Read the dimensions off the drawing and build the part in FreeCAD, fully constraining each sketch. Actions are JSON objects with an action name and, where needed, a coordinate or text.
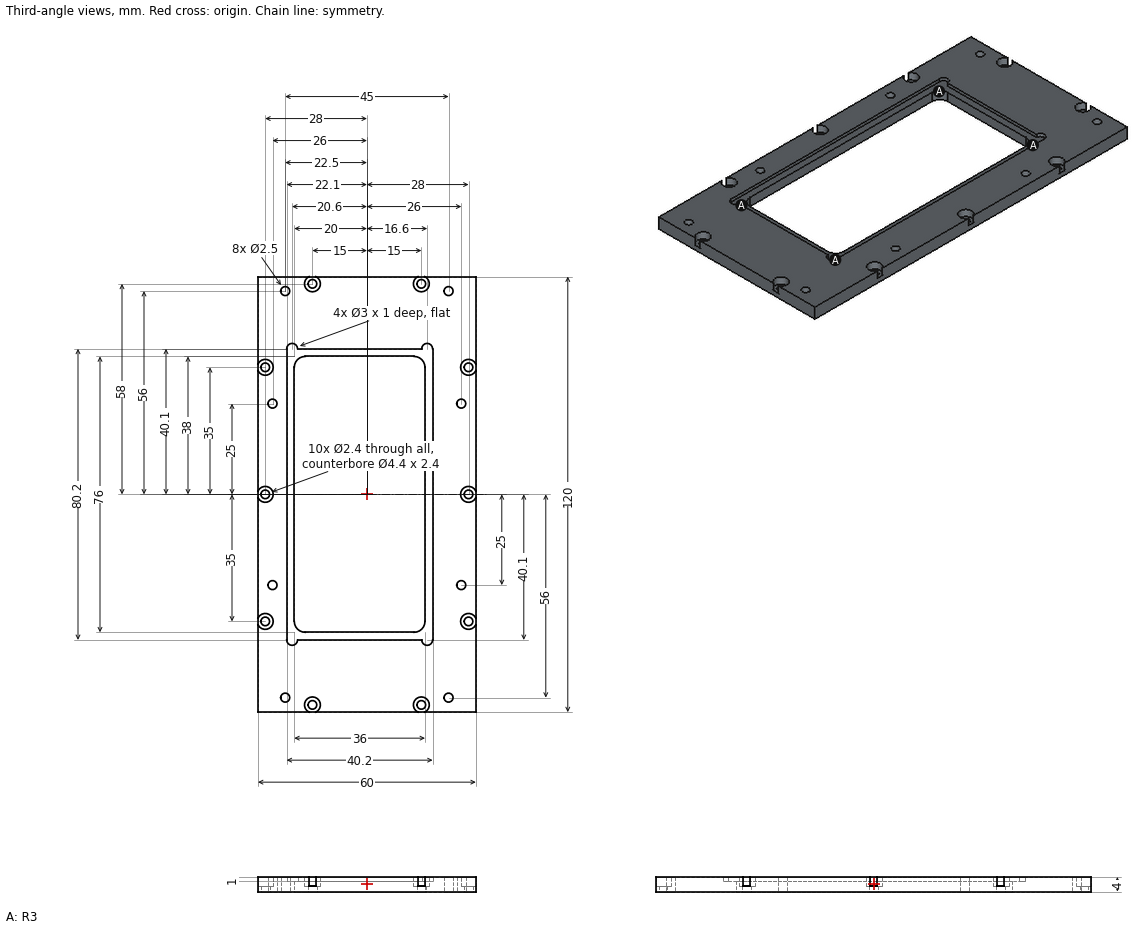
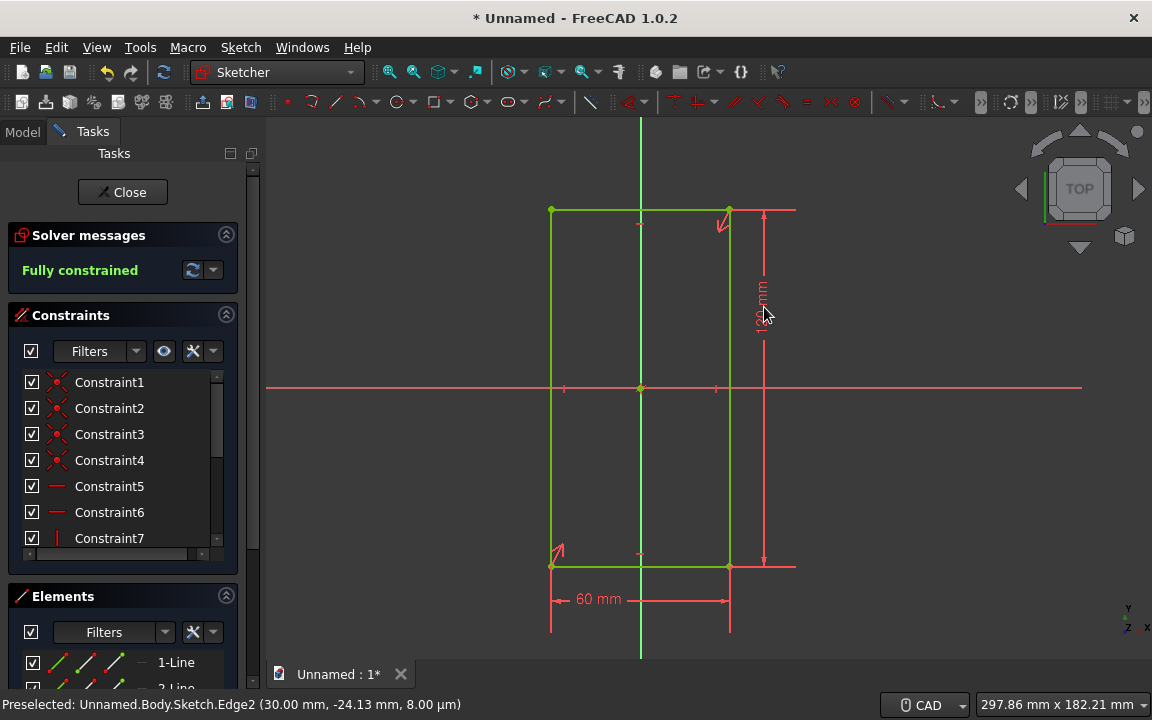
{"action": "left_click", "coordinate": [123, 192]}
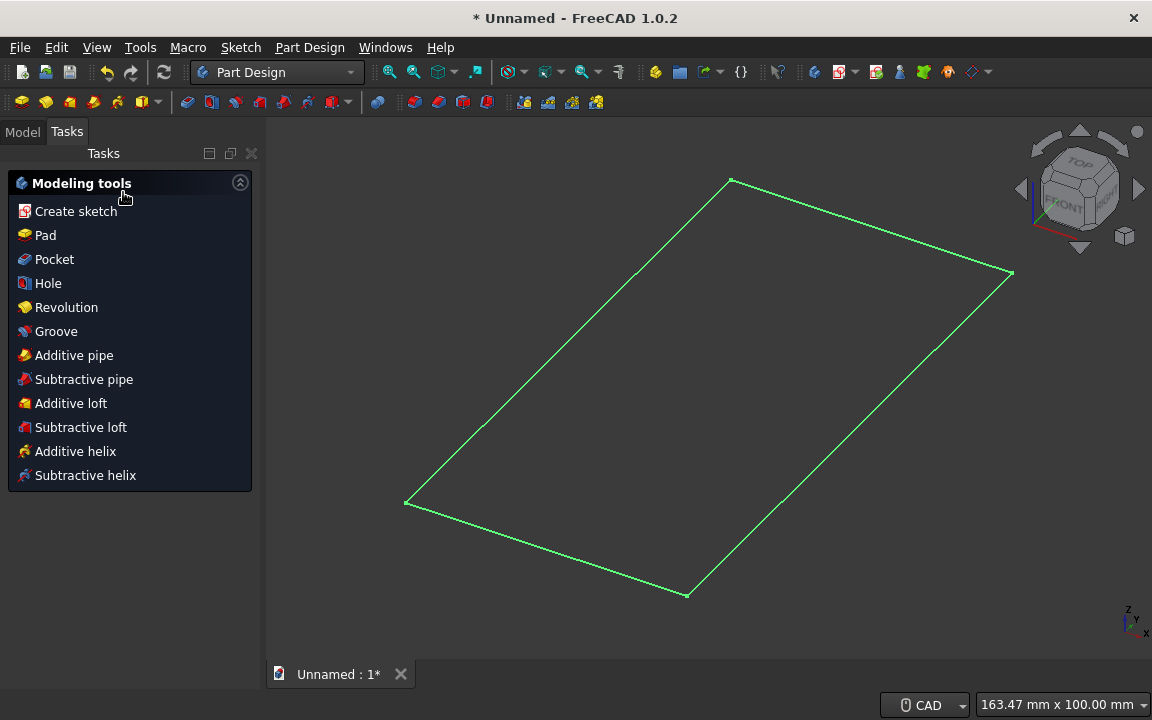
{"action": "left_click", "coordinate": [22, 102]}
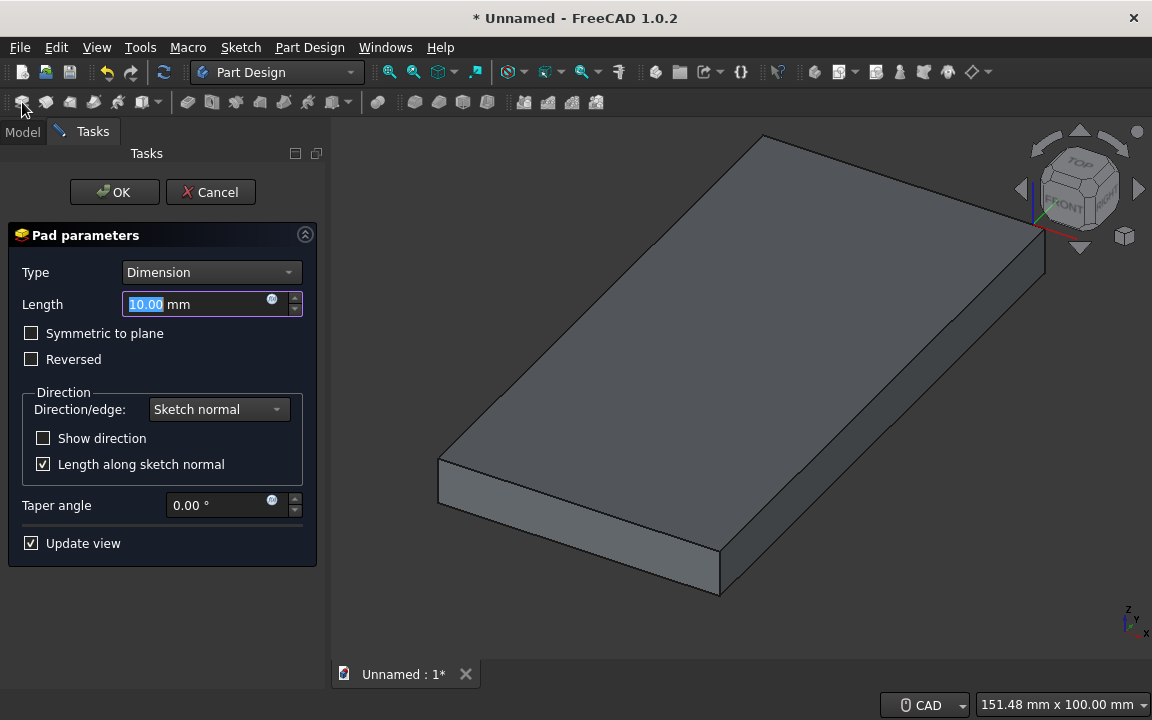
{"action": "type", "text": "4"}
{"action": "key", "text": "Tab"}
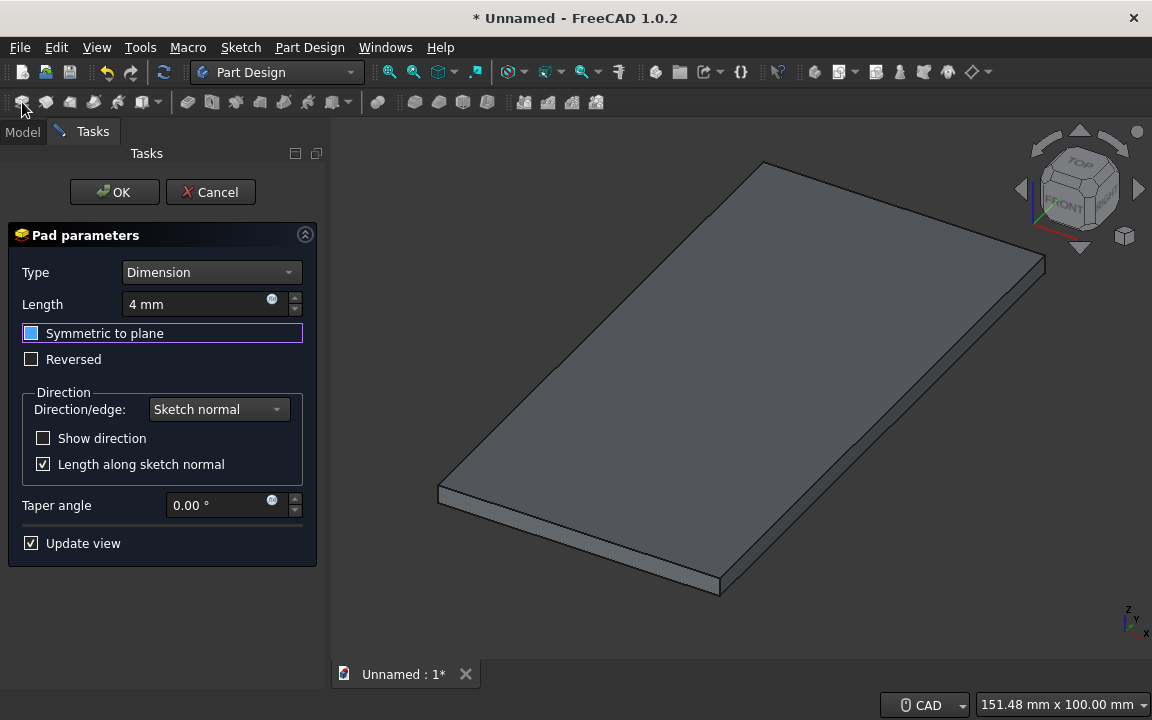
{"action": "left_click", "coordinate": [30, 333]}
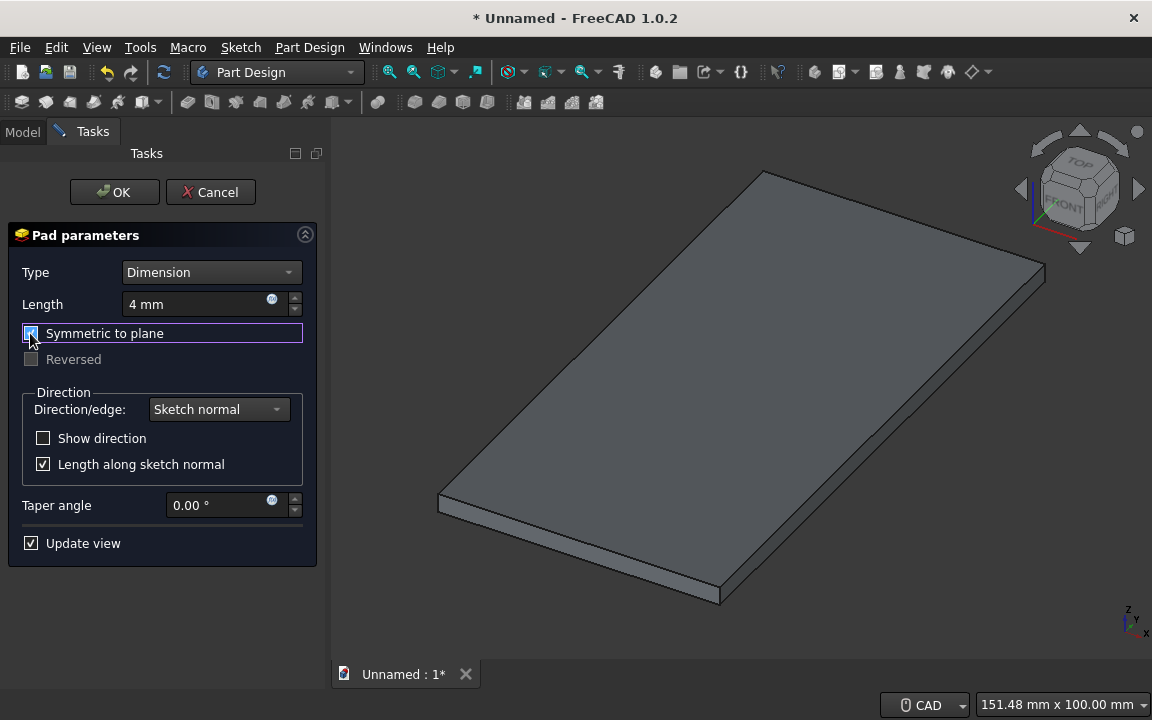
{"action": "left_click", "coordinate": [115, 192]}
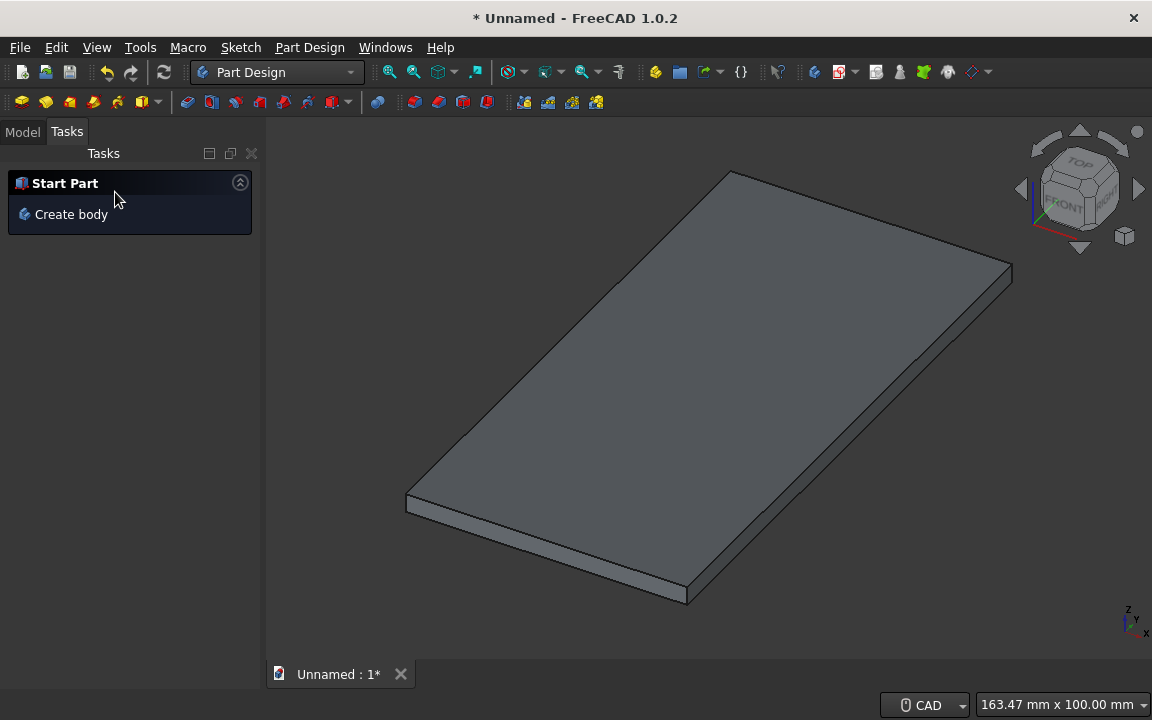
{"action": "left_click", "coordinate": [755, 332]}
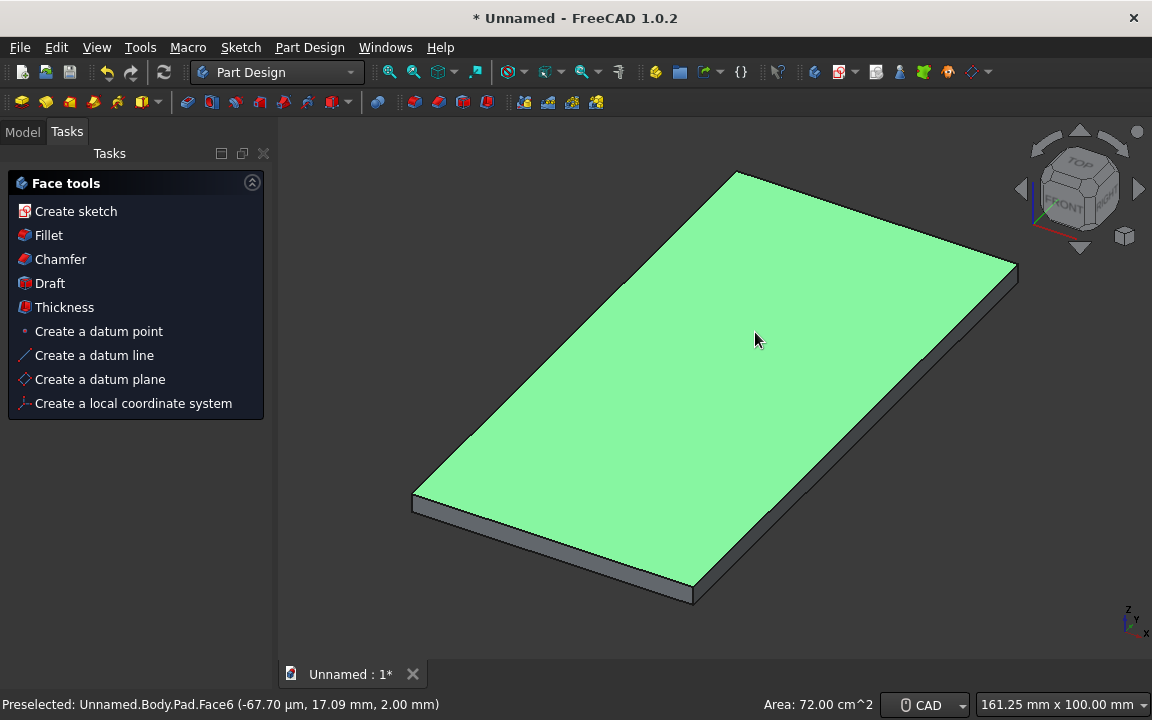
{"action": "left_click", "coordinate": [840, 72]}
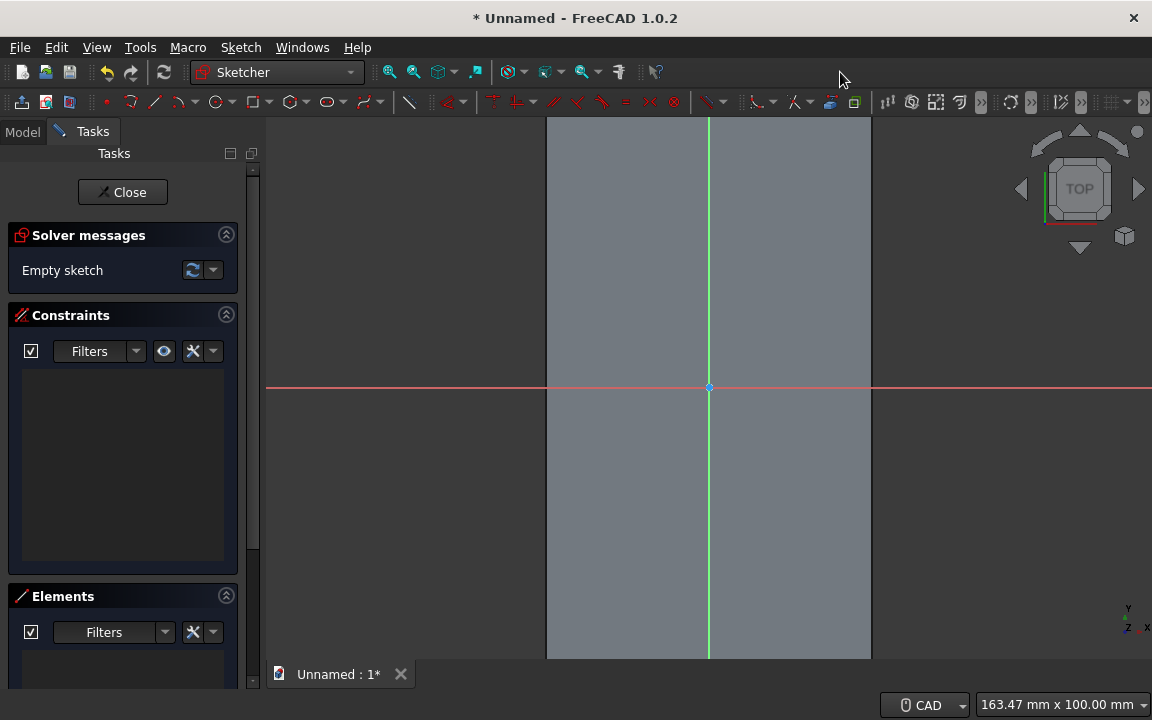
{"action": "key", "text": "g r"}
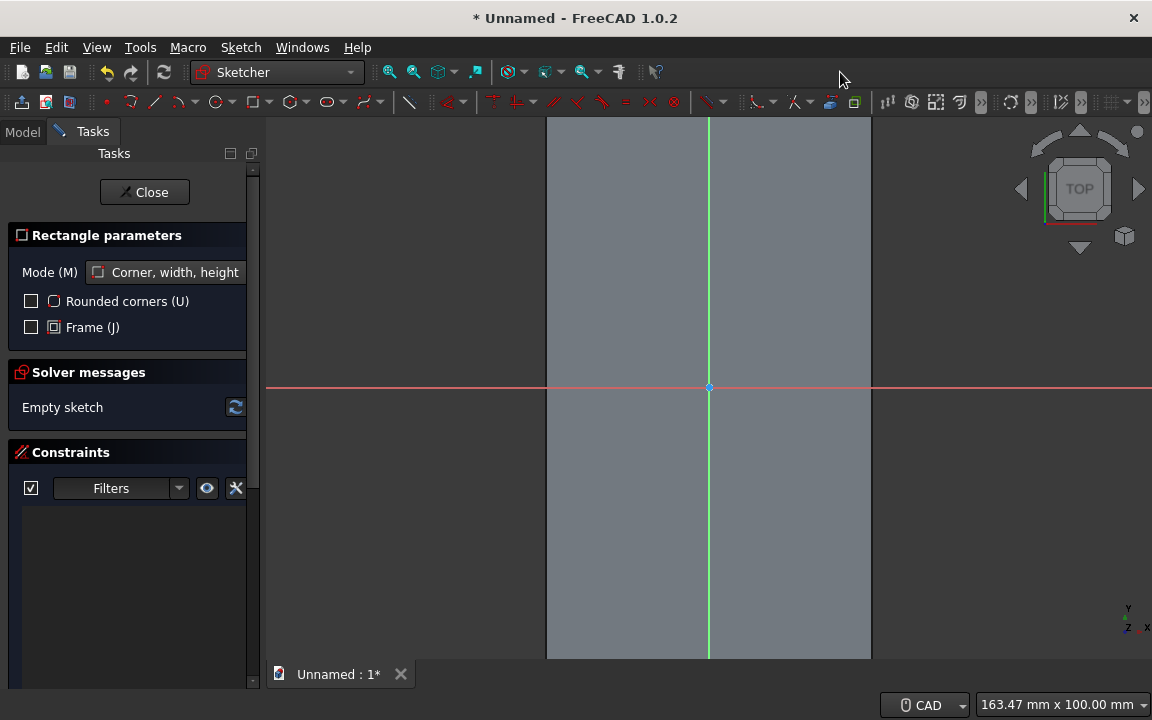
{"action": "left_click", "coordinate": [601, 182]}
{"action": "left_click", "coordinate": [796, 594]}
{"action": "key", "text": "Escape"}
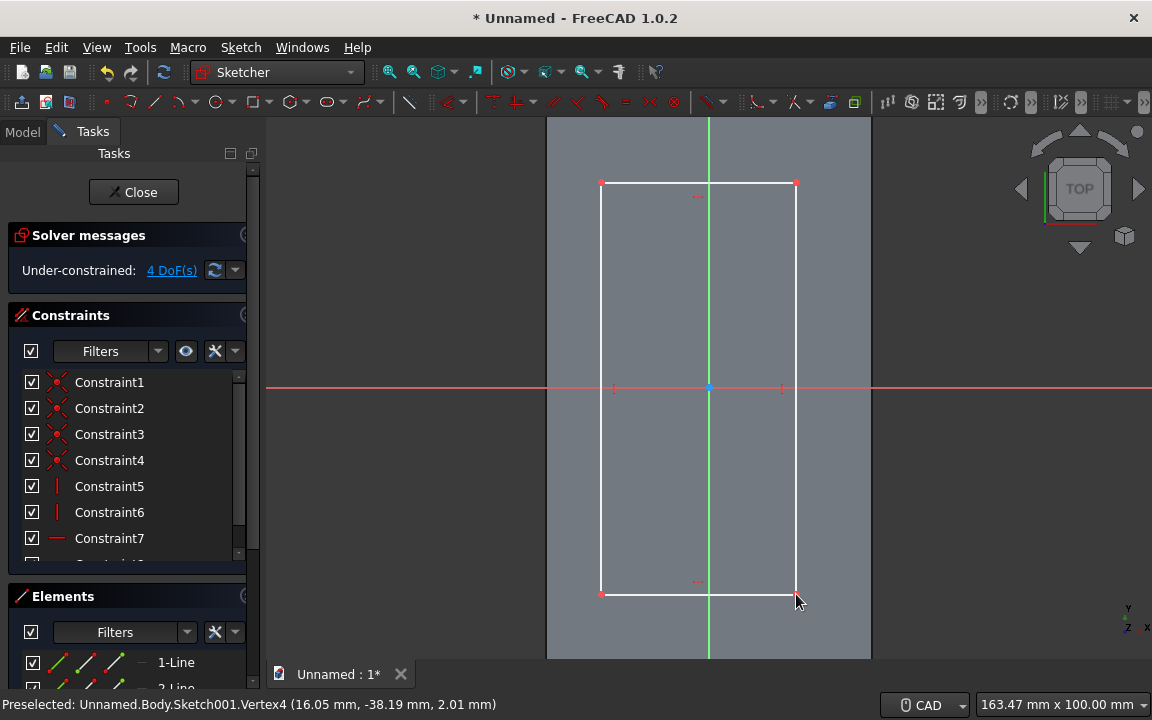
{"action": "key", "text": "d"}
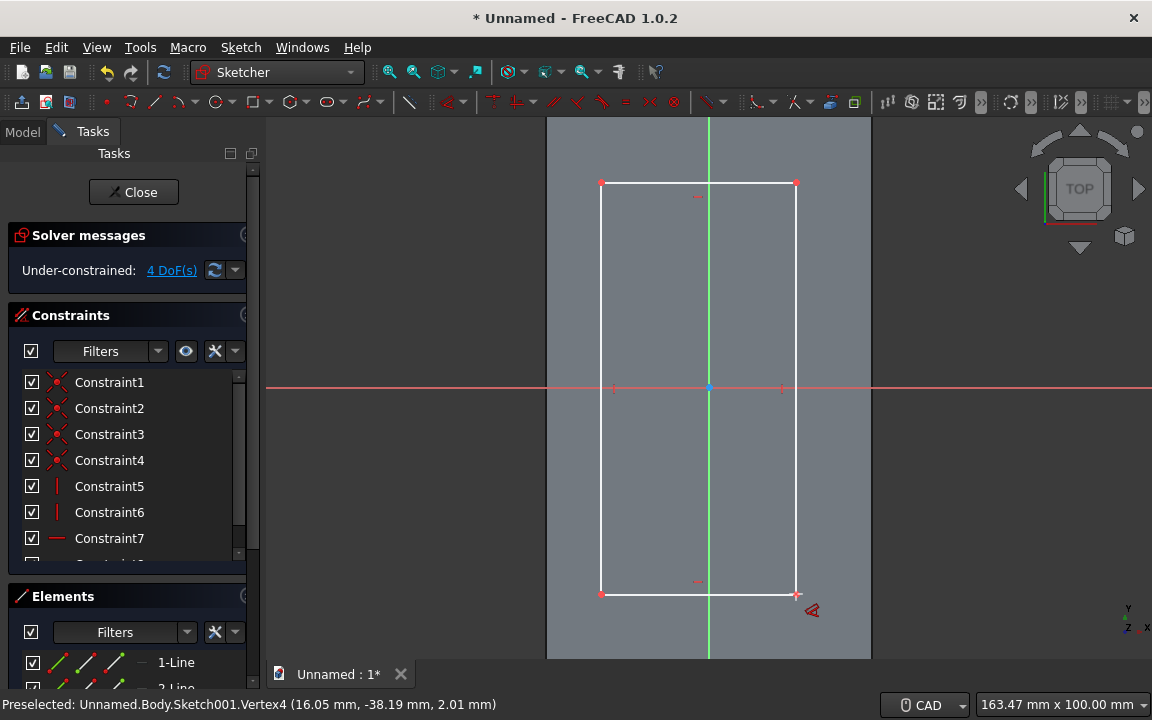
{"action": "left_click", "coordinate": [601, 307]}
{"action": "left_click", "coordinate": [567, 294]}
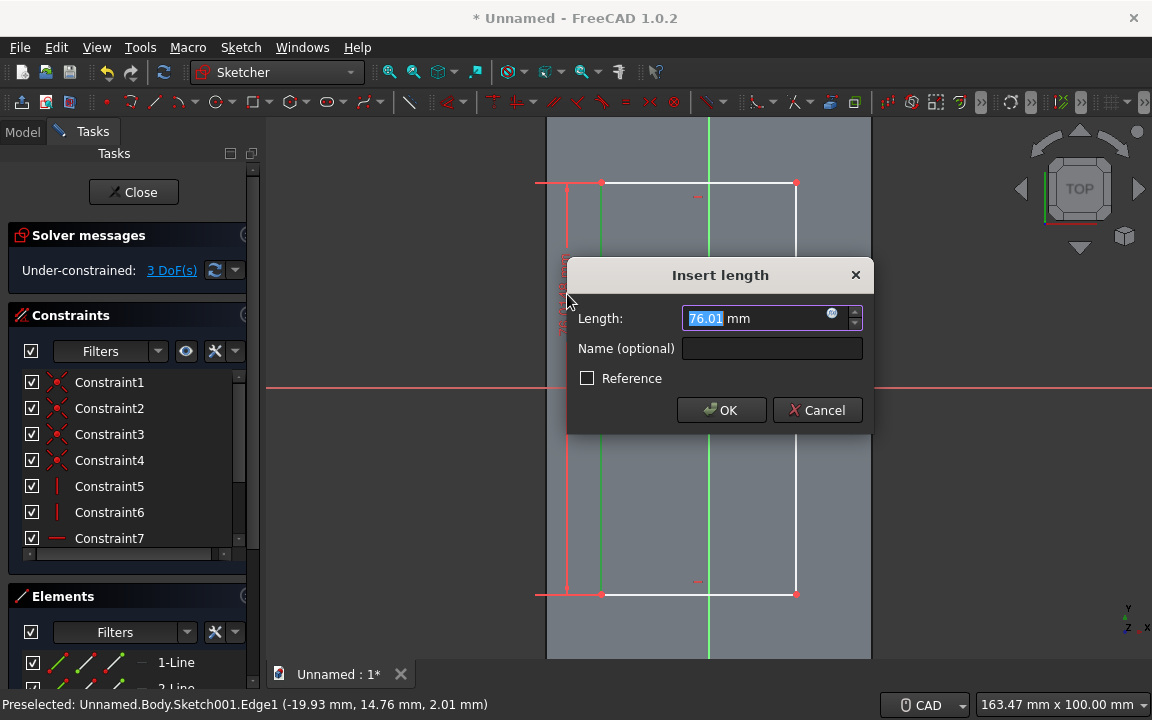
{"action": "type", "text": "76"}
{"action": "key", "text": "Return"}